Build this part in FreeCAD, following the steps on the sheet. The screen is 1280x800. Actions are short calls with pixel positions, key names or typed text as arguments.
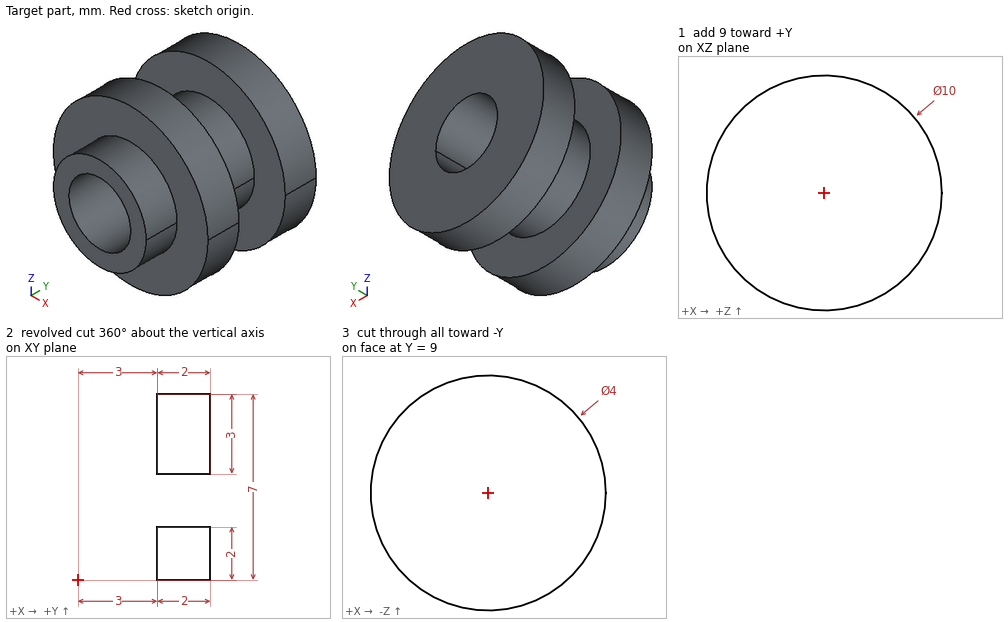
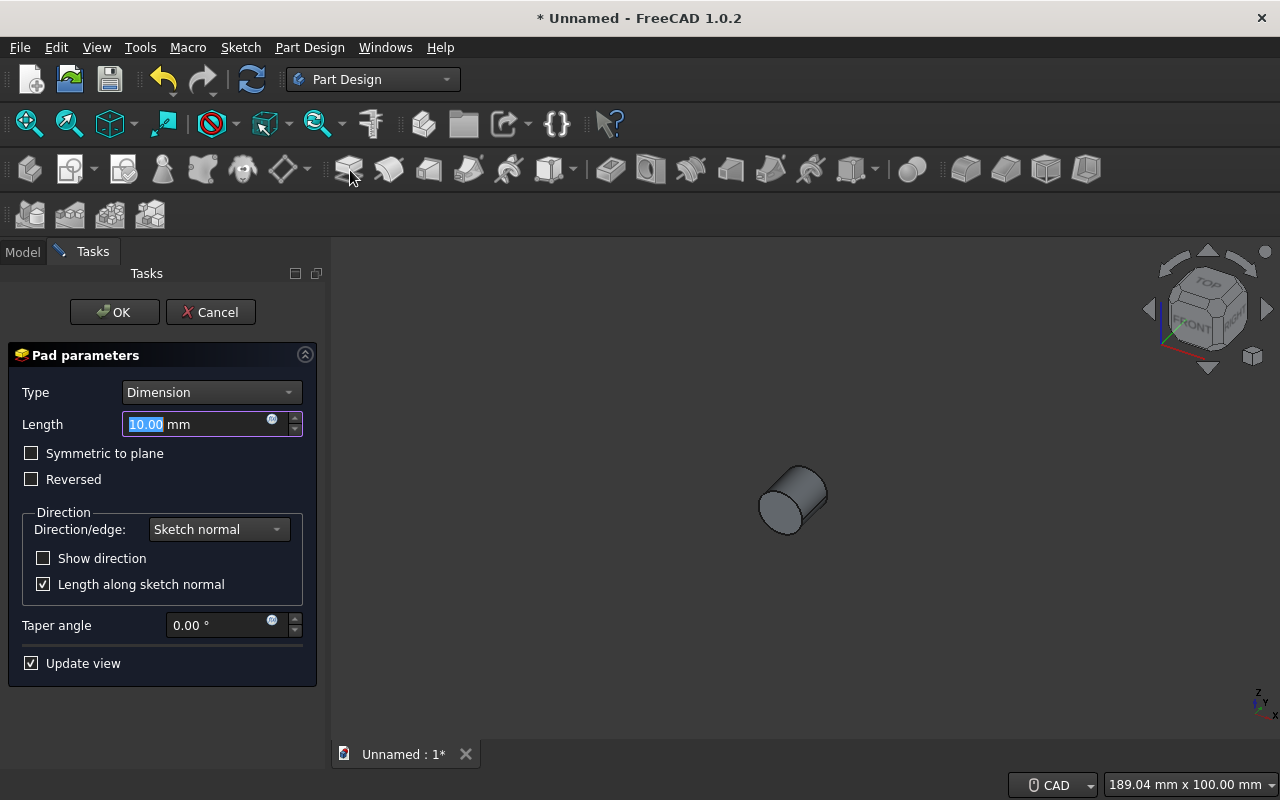
text(9)
key(Tab)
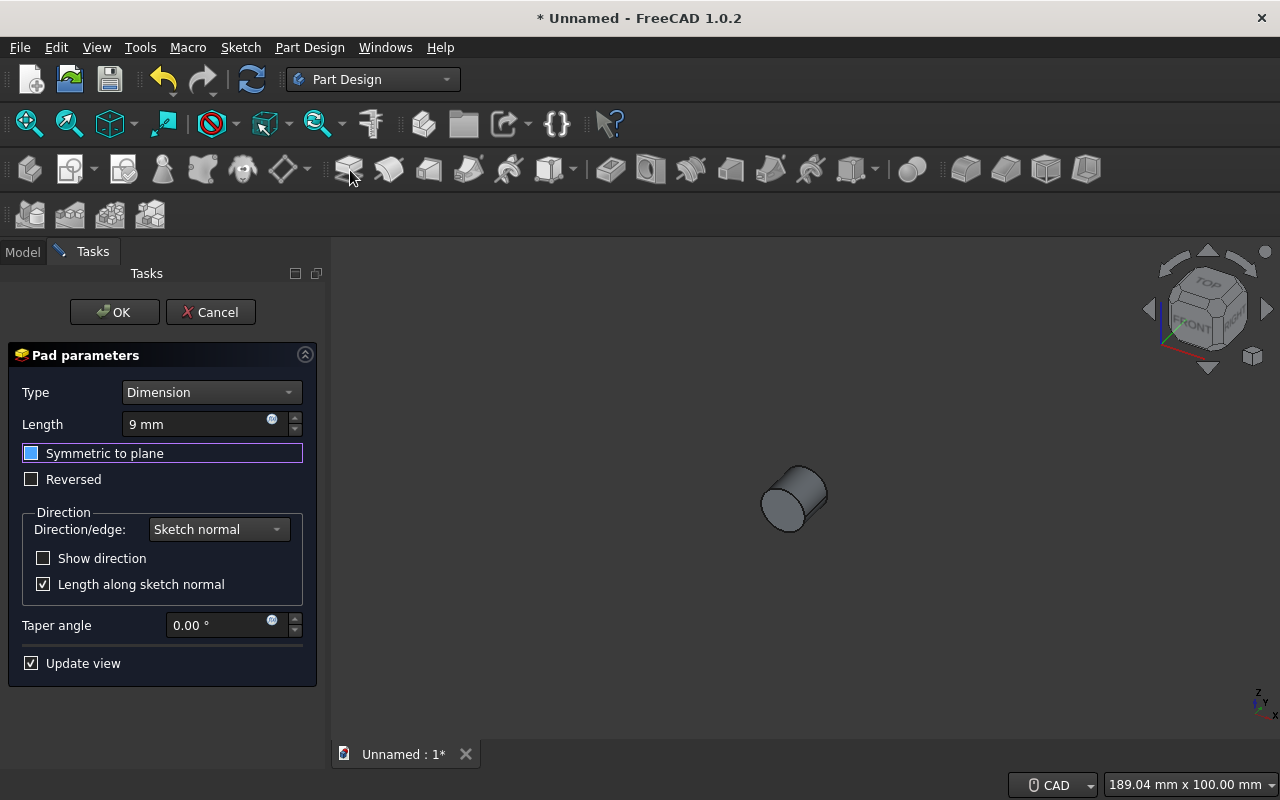
click(30, 479)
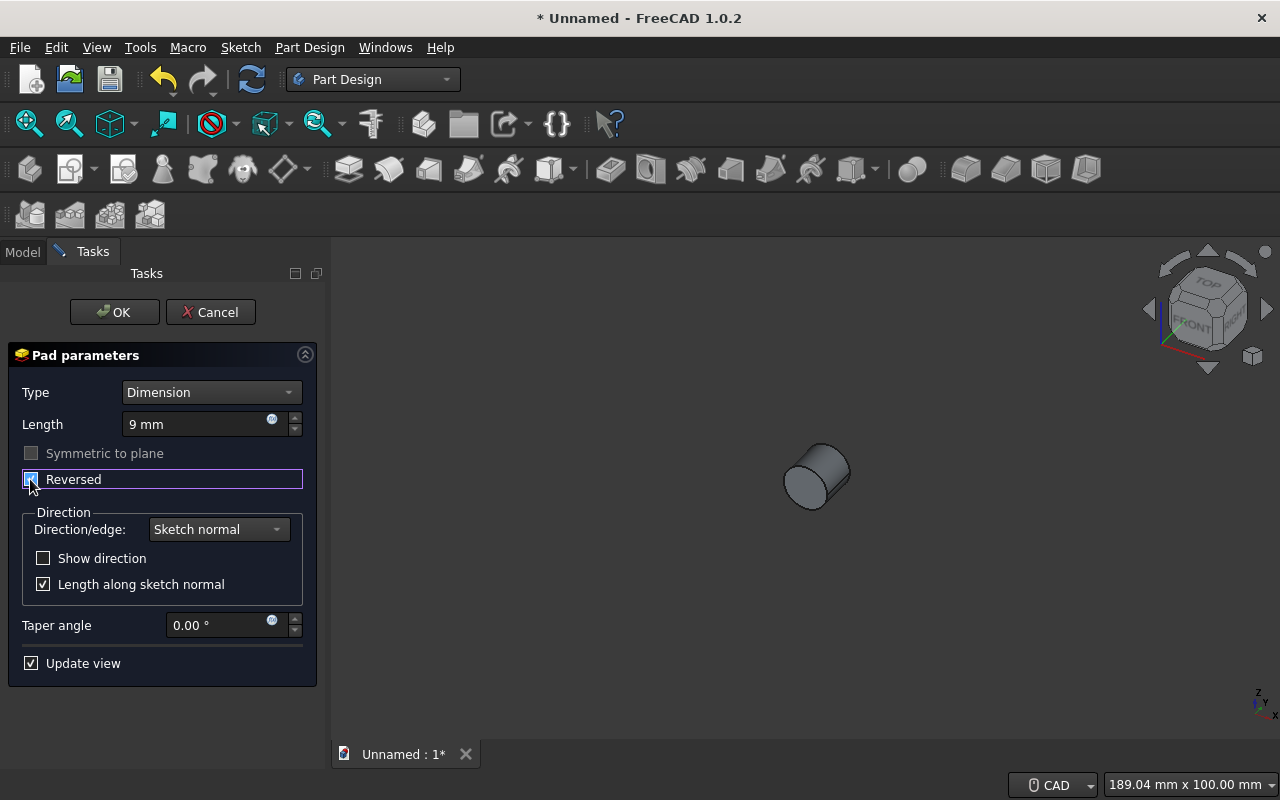
click(115, 312)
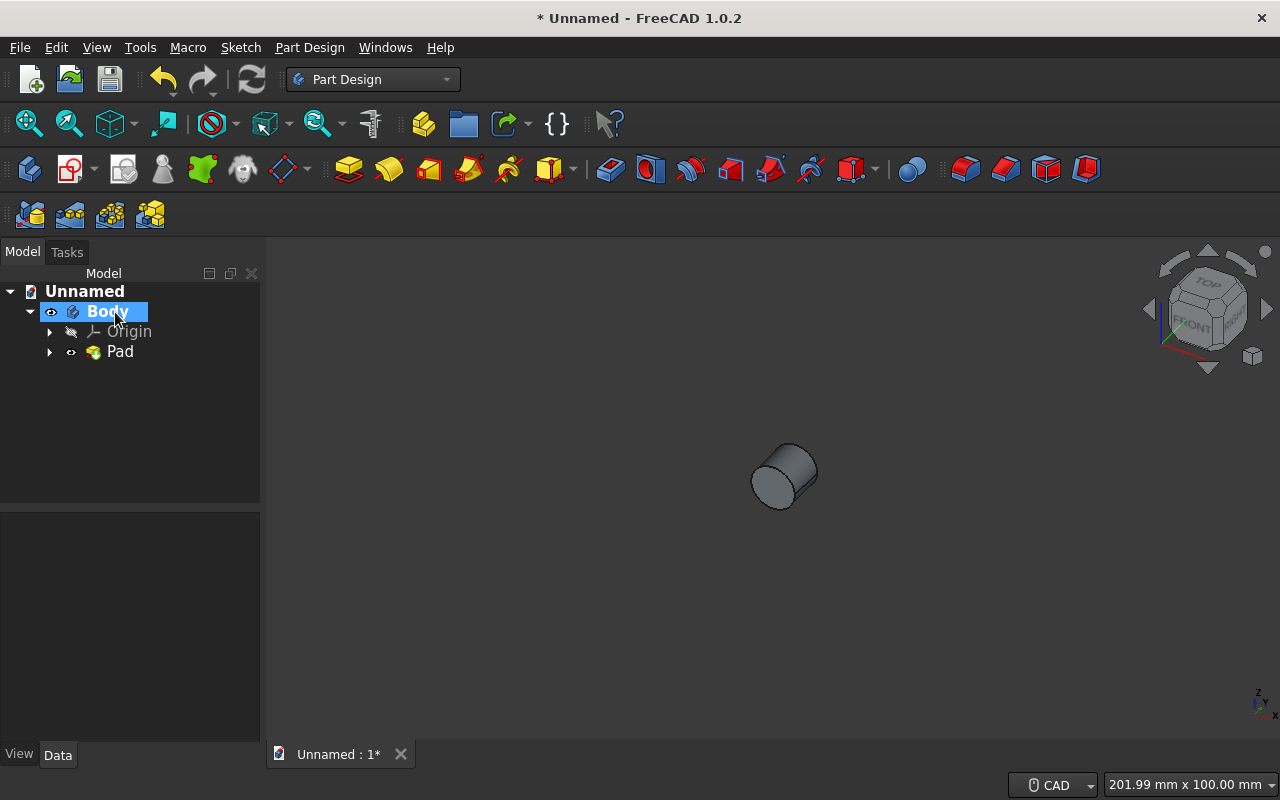
click(30, 124)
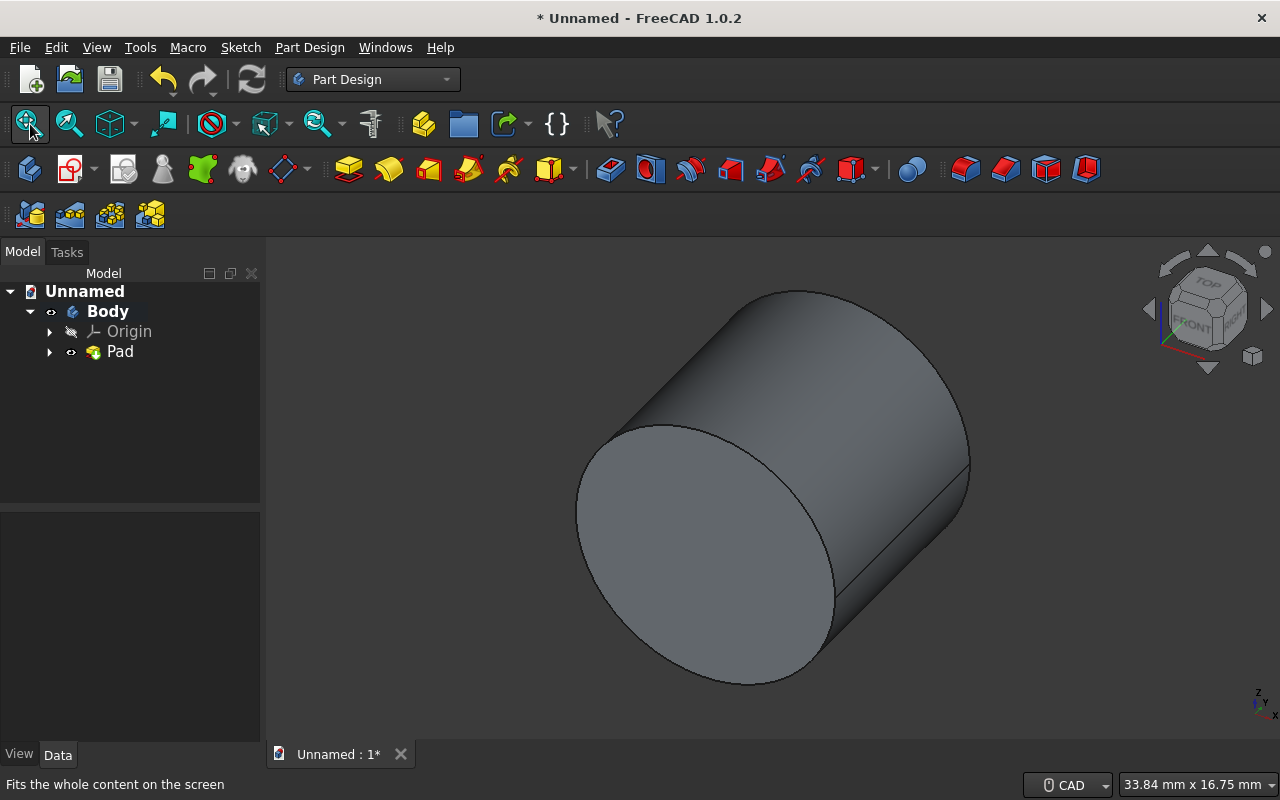
click(70, 170)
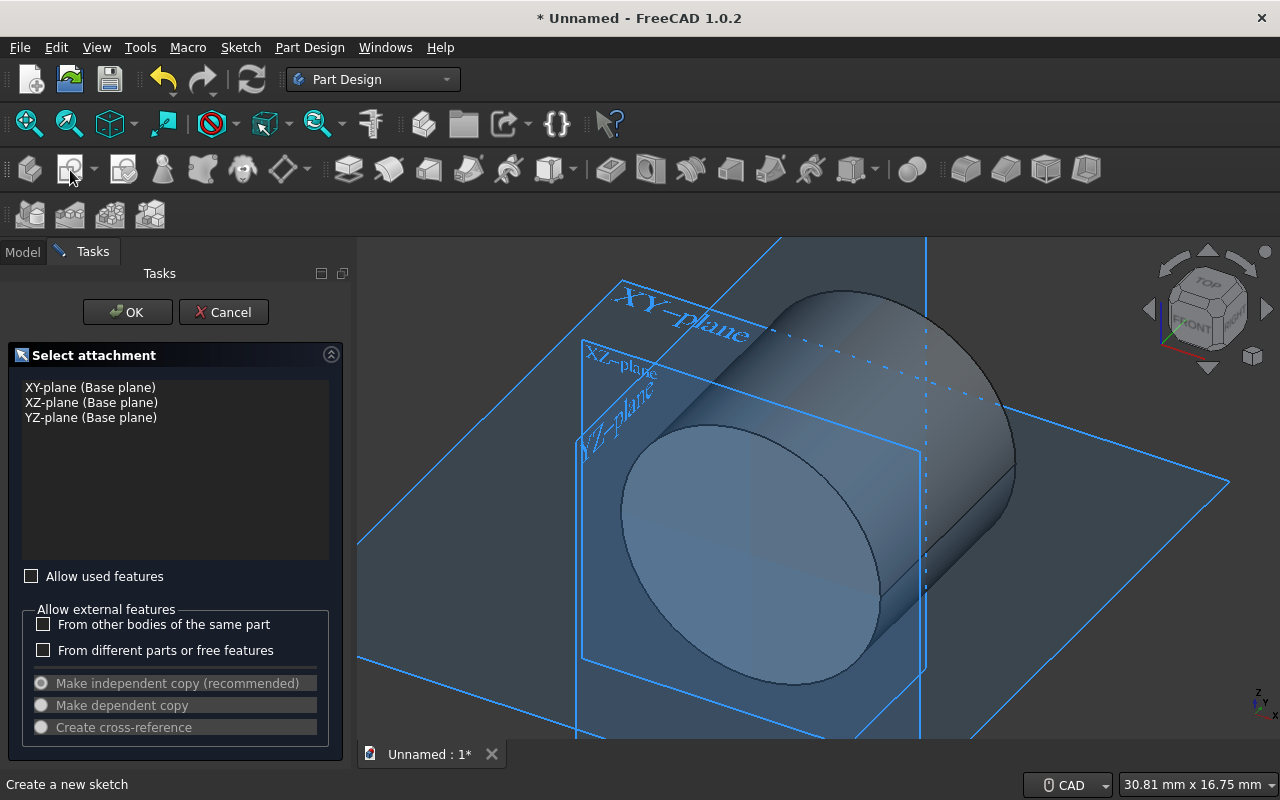
click(82, 388)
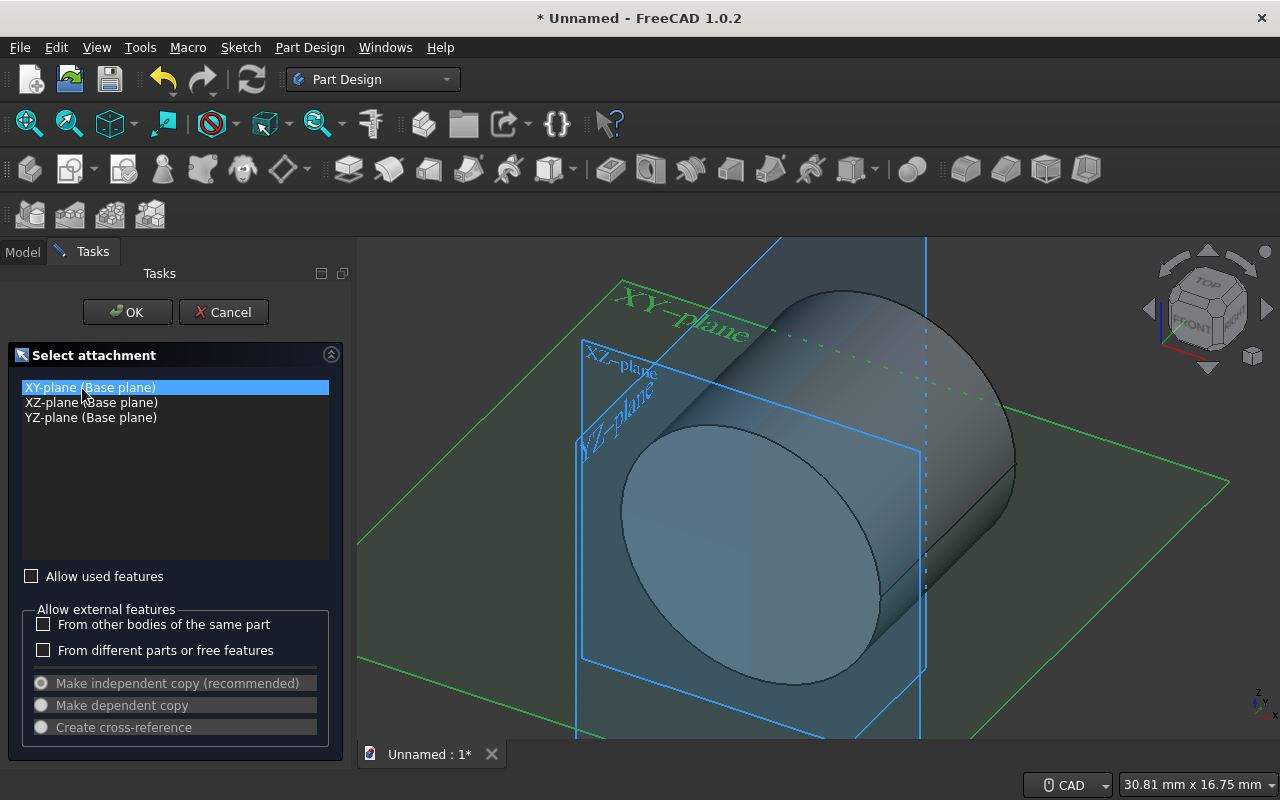
click(128, 312)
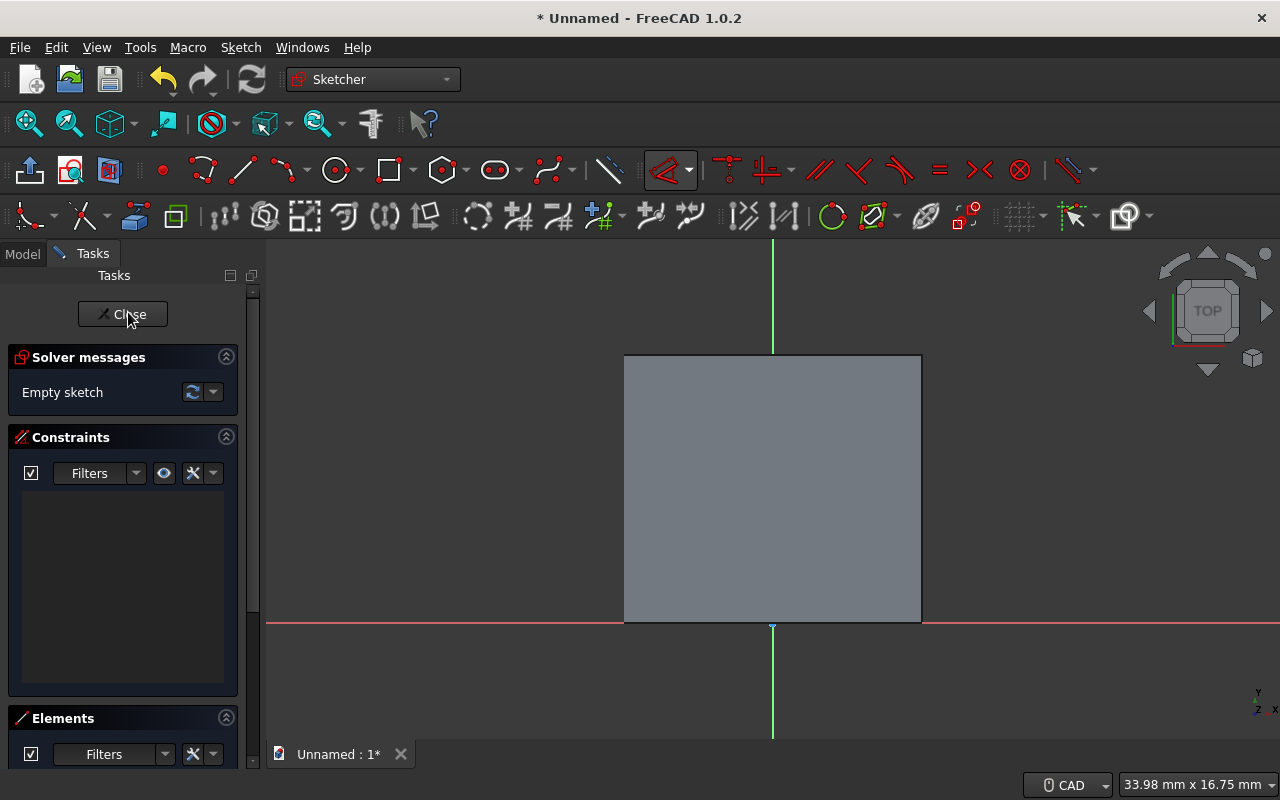
click(110, 170)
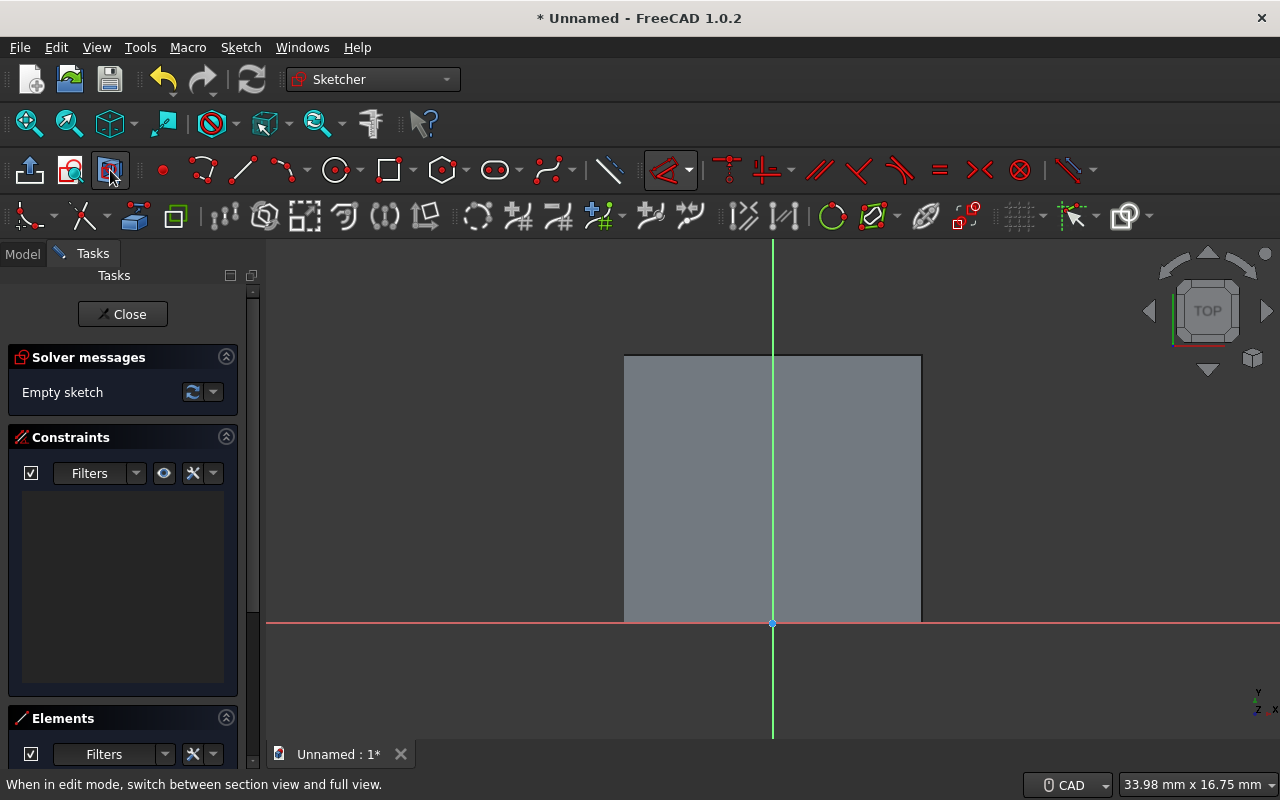
scroll(1115, 580, up, 2)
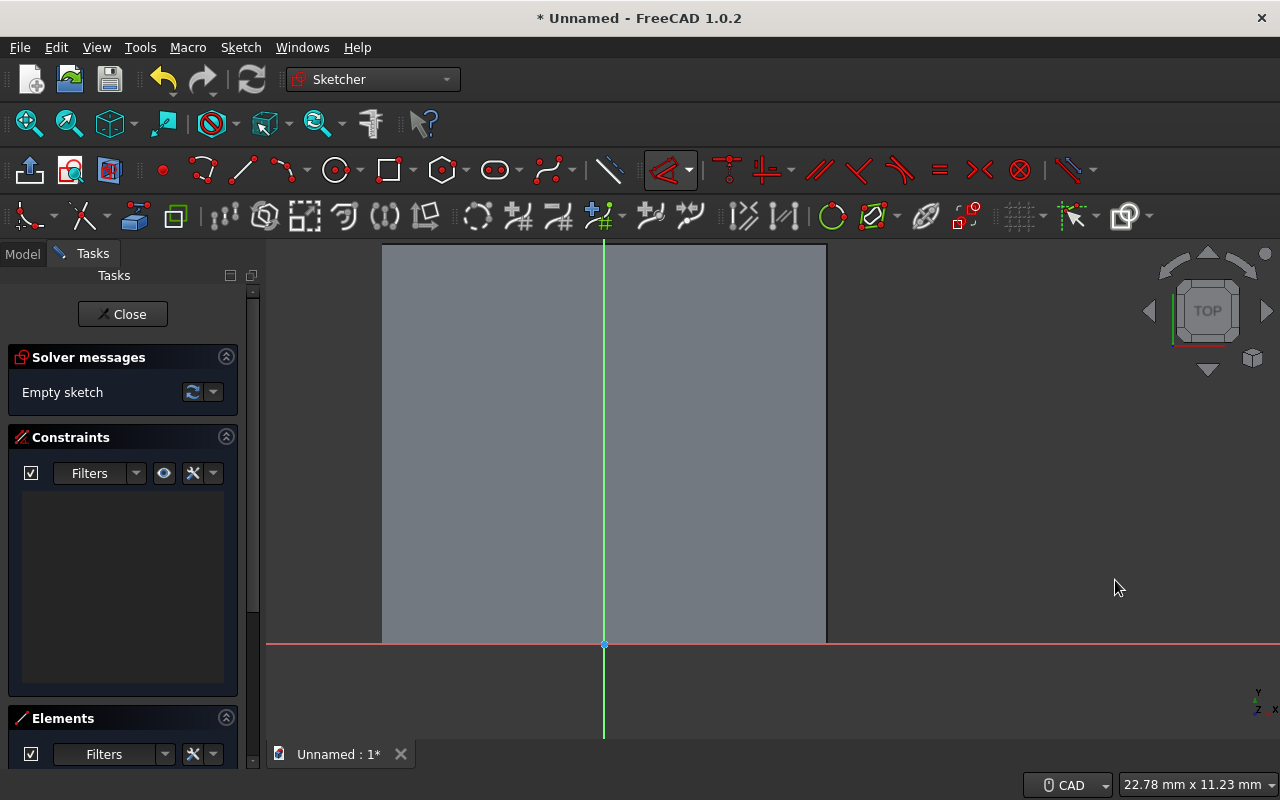
click(390, 170)